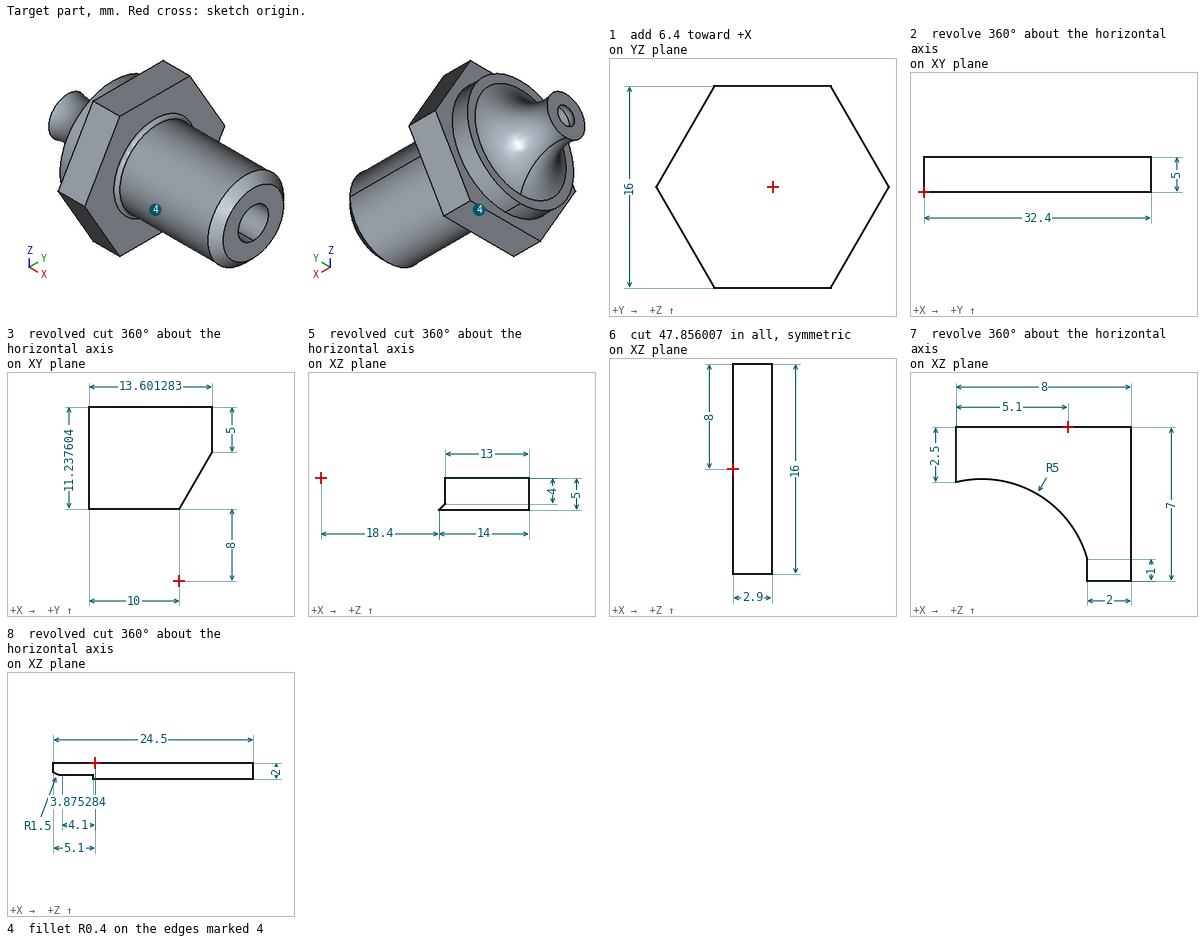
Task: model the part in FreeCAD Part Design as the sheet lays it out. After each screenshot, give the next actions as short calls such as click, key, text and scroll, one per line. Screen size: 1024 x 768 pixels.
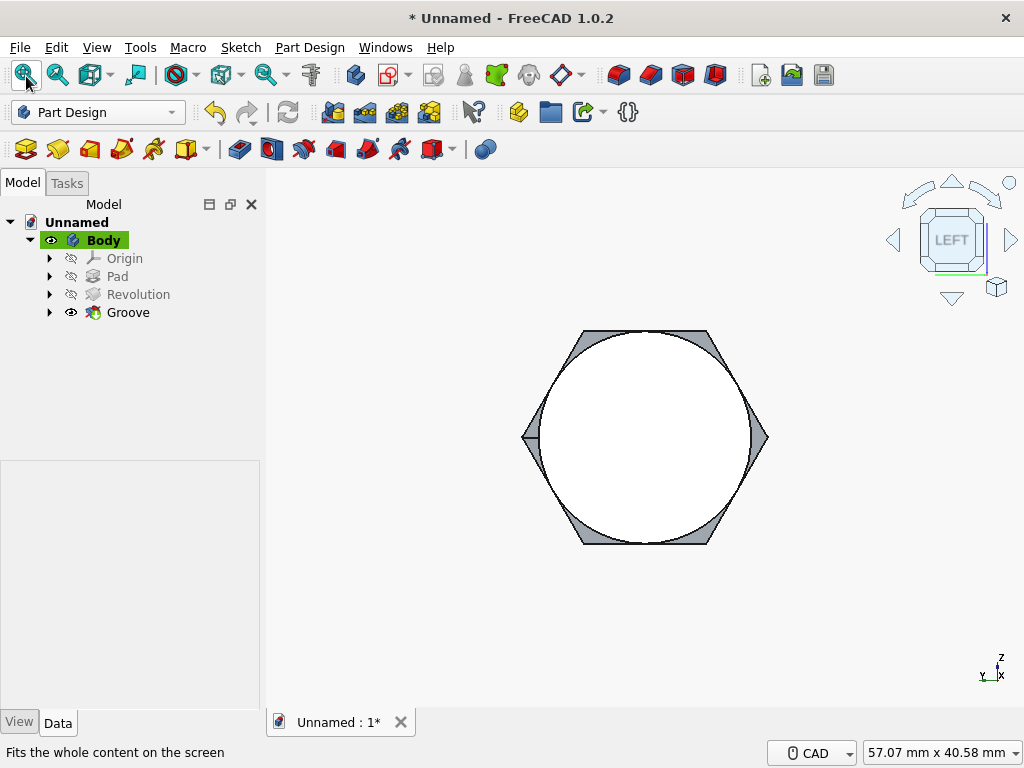
key(v)
key(3)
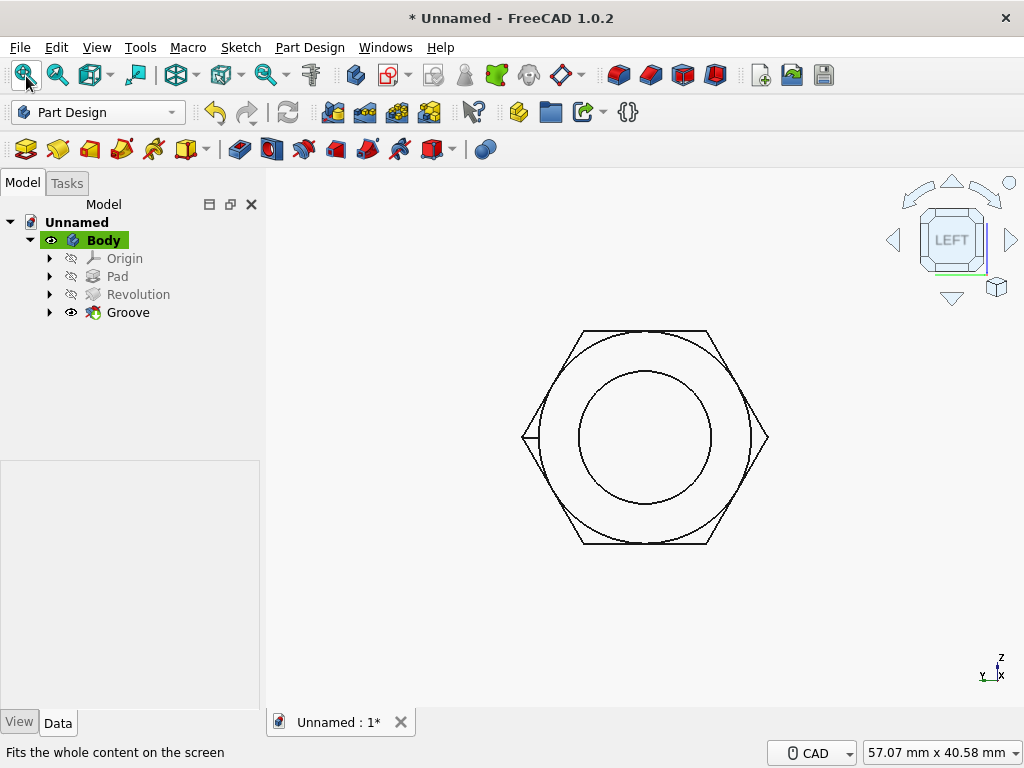
key(0)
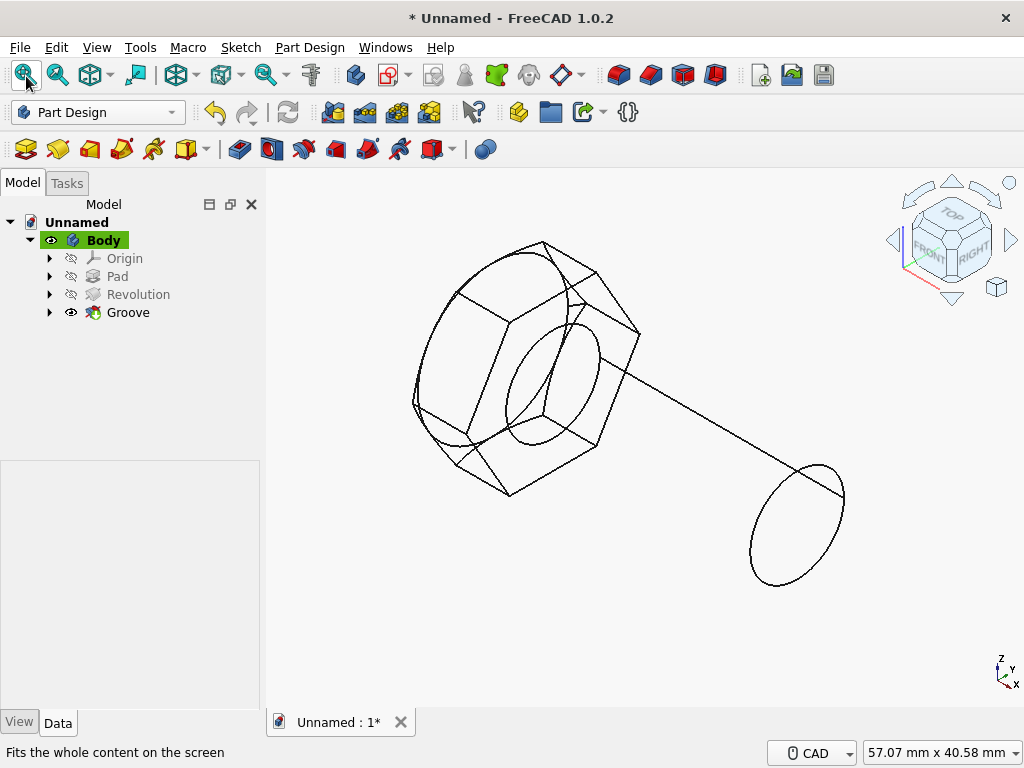
click(506, 410)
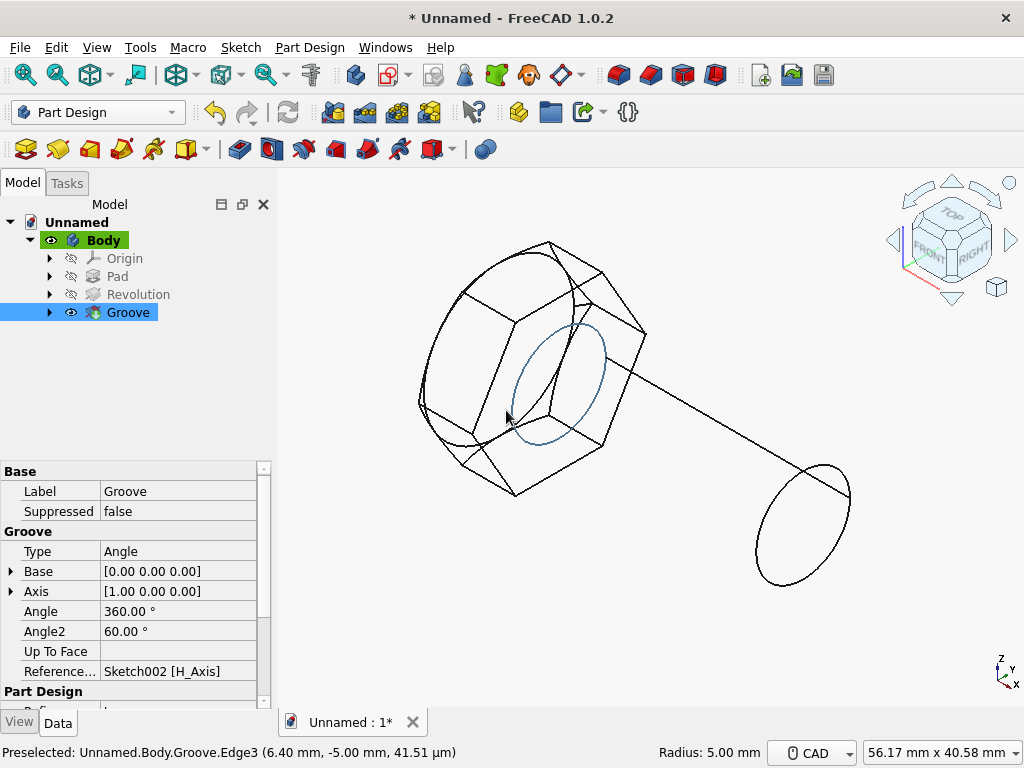
key(v)
key(1)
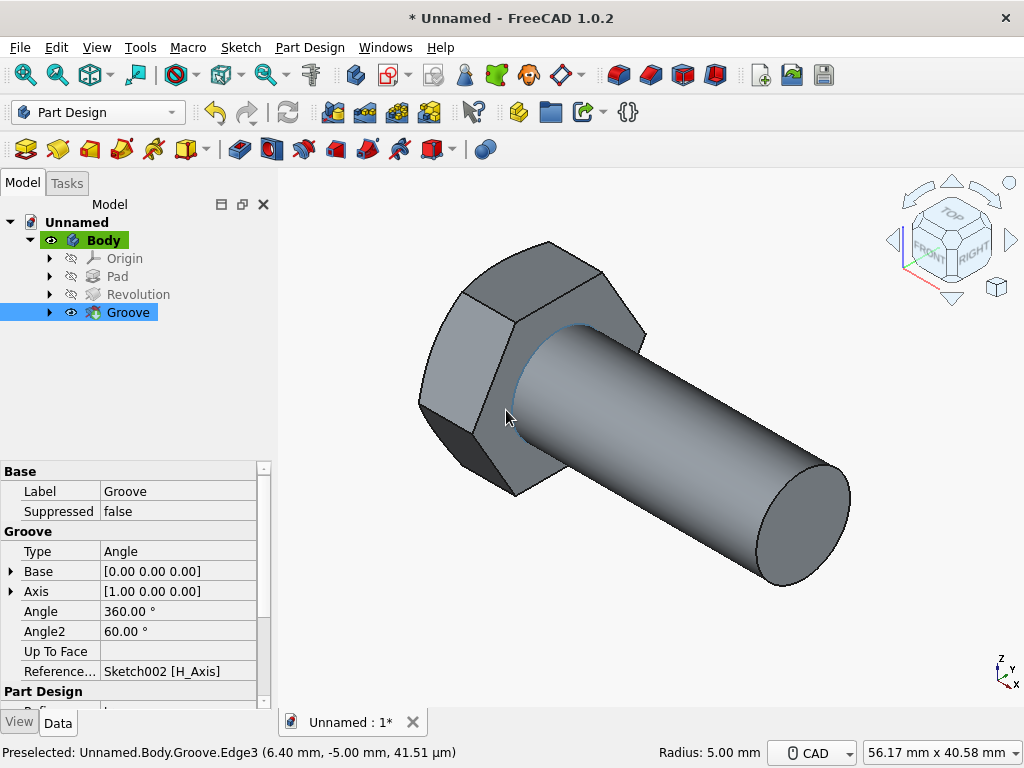
click(620, 76)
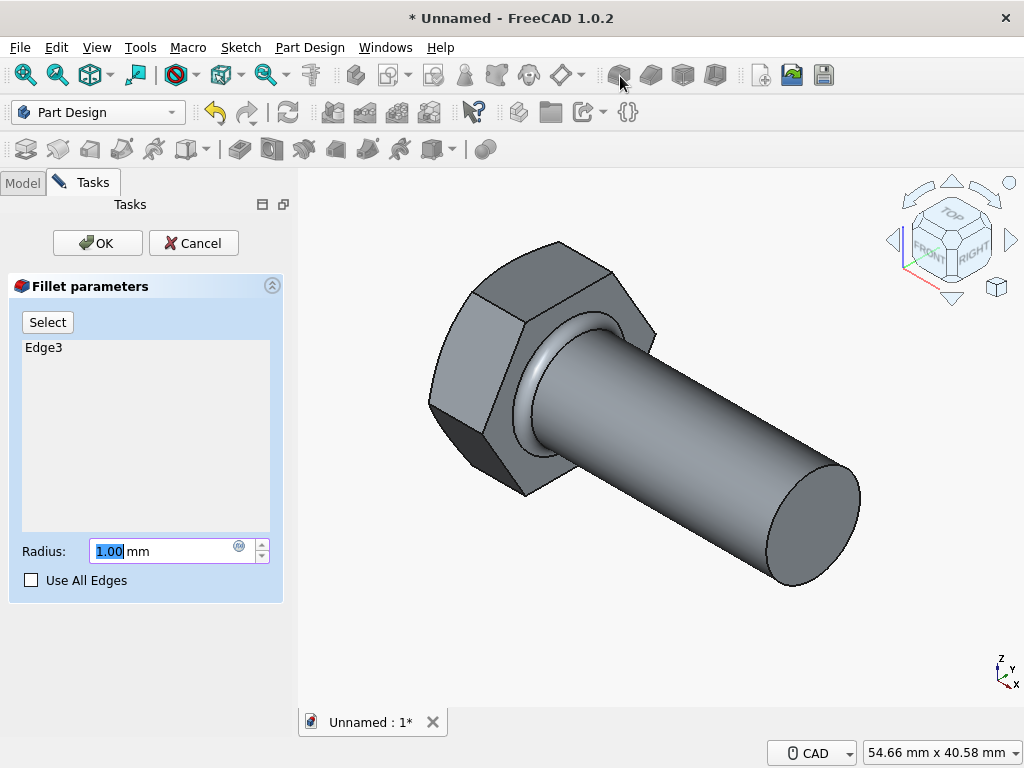
text(0.4)
key(Tab)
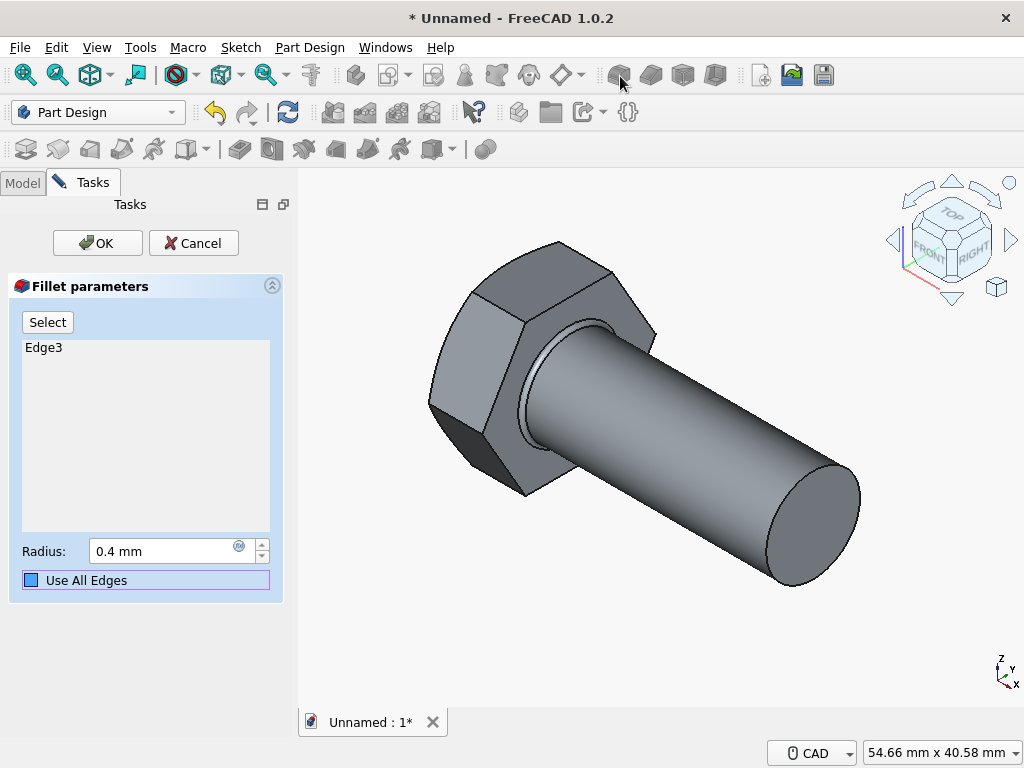
click(98, 243)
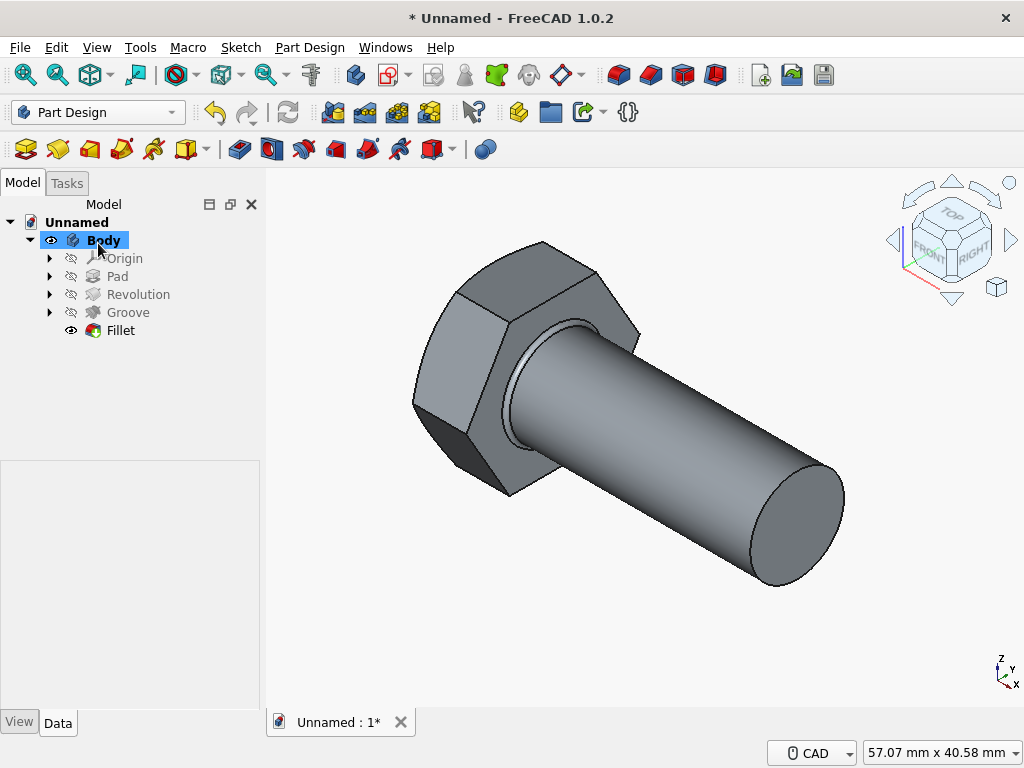
click(388, 76)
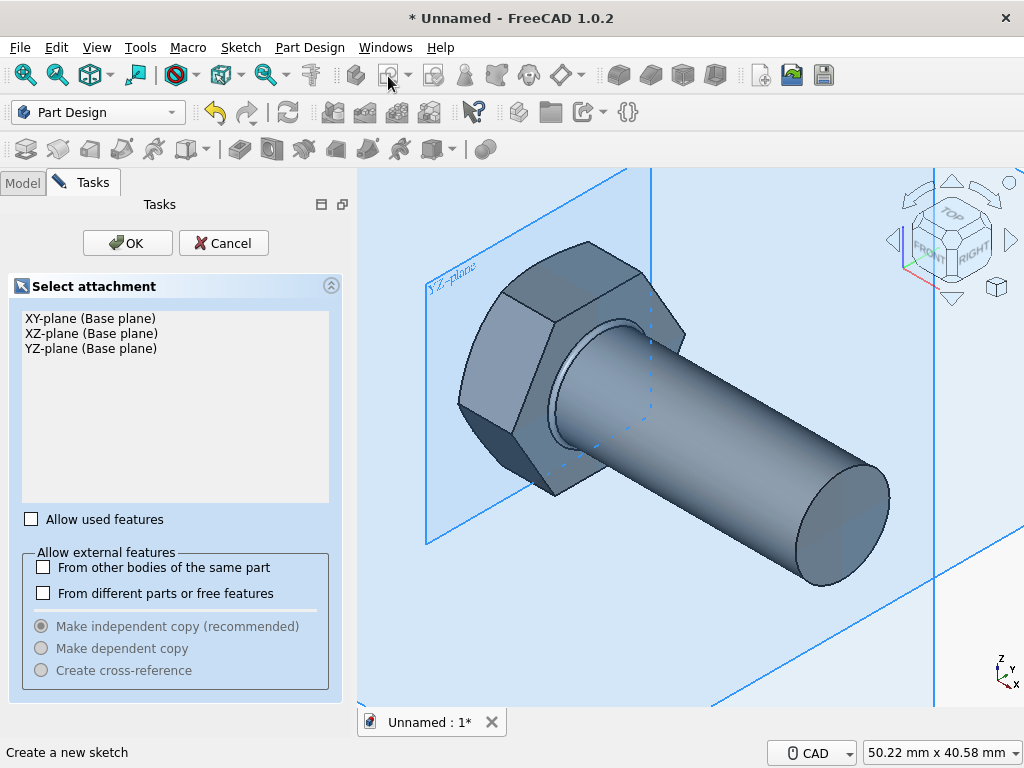
click(82, 334)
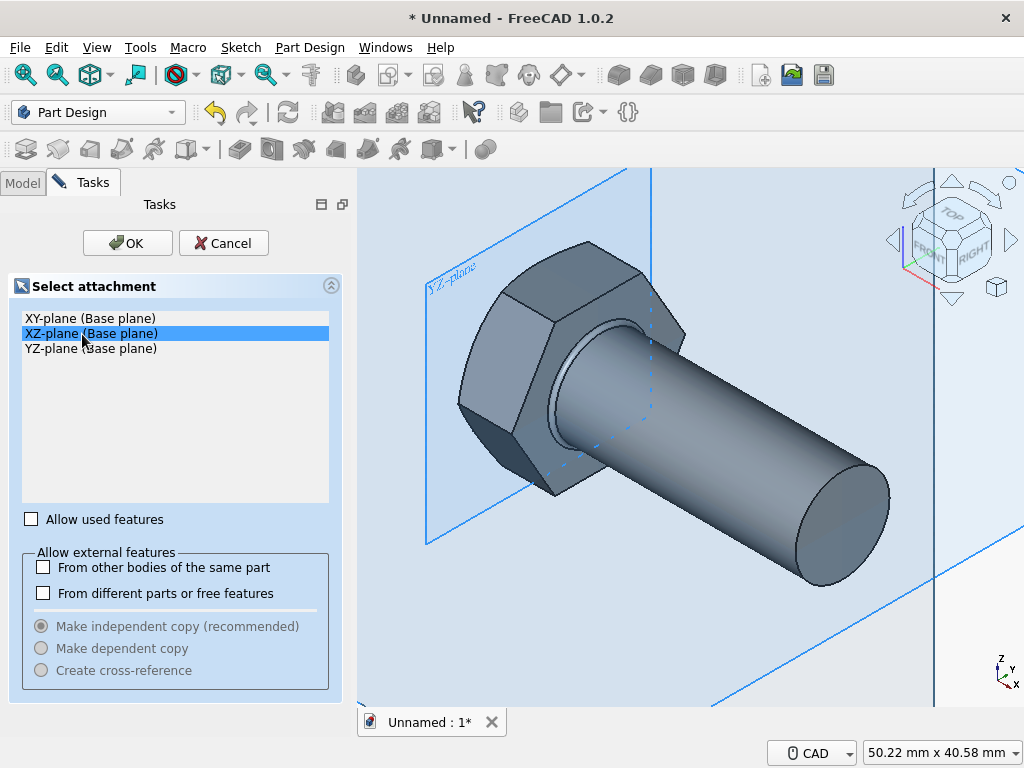
click(128, 243)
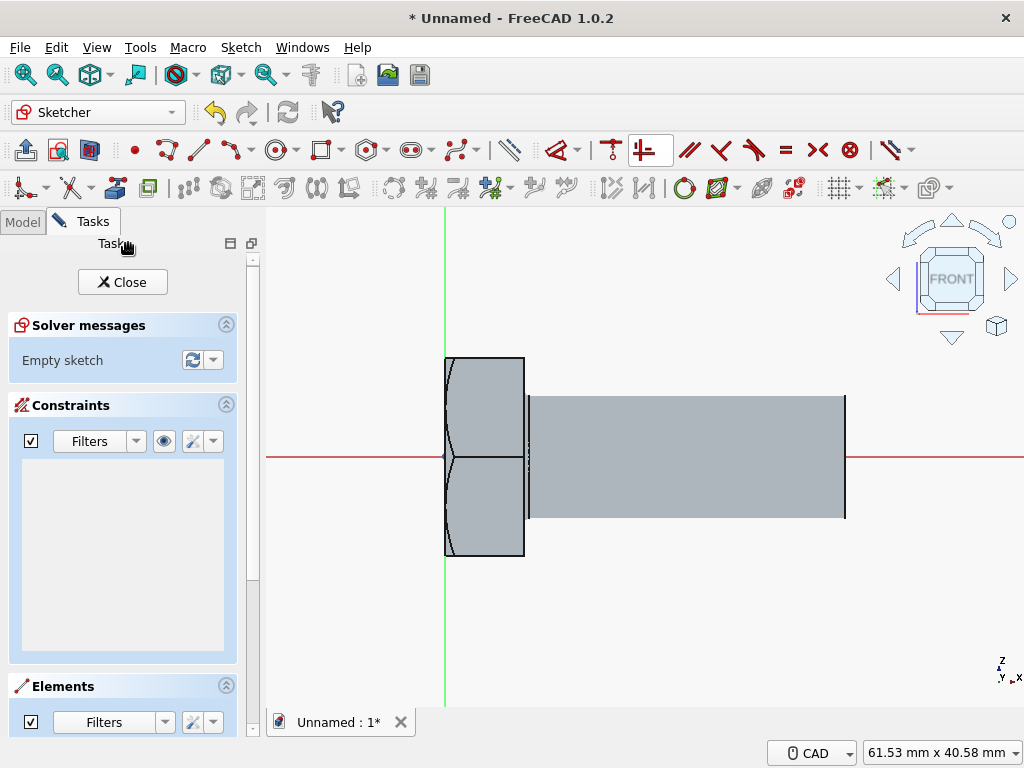
click(90, 150)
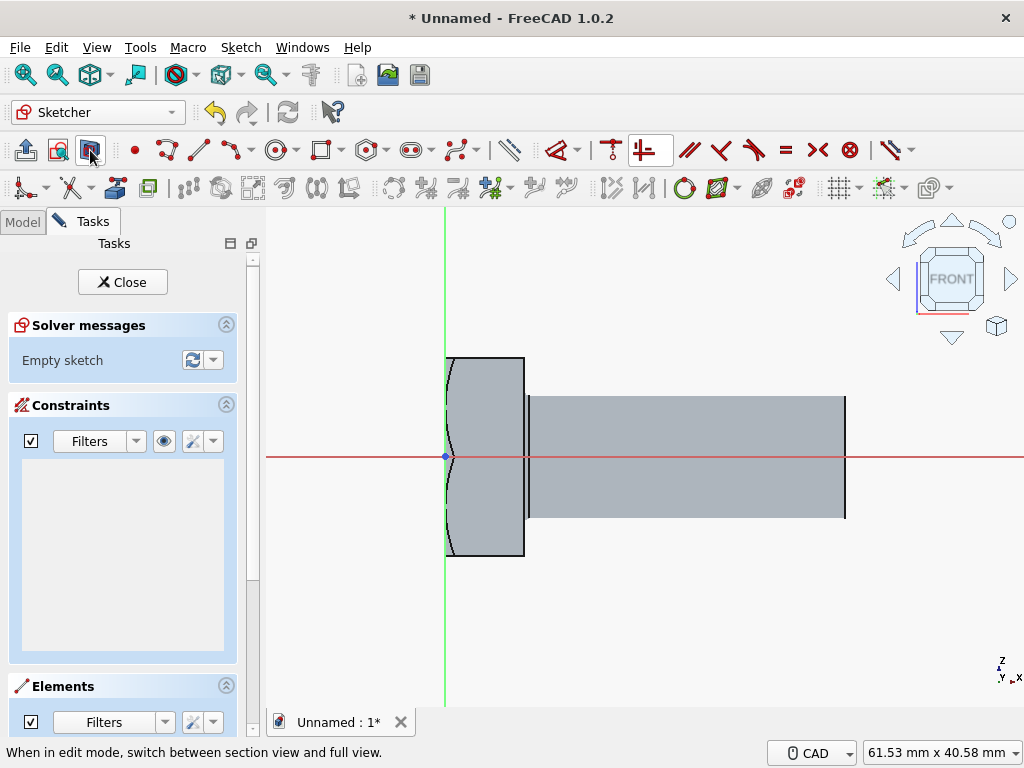
scroll(294, 318, down, 1)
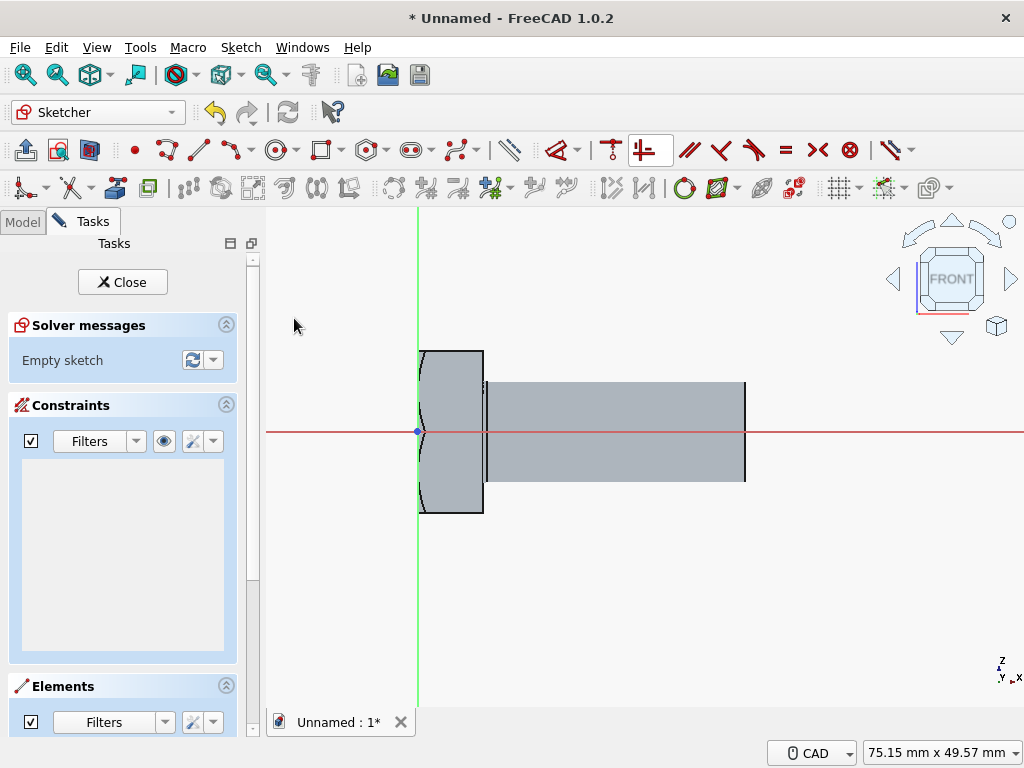
click(168, 150)